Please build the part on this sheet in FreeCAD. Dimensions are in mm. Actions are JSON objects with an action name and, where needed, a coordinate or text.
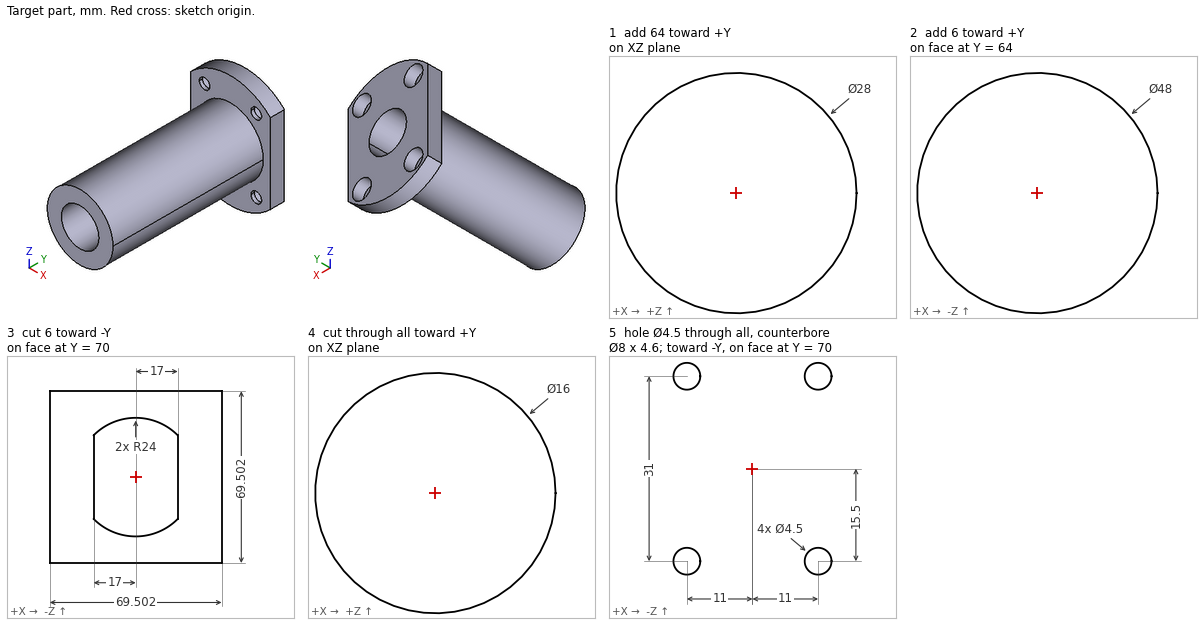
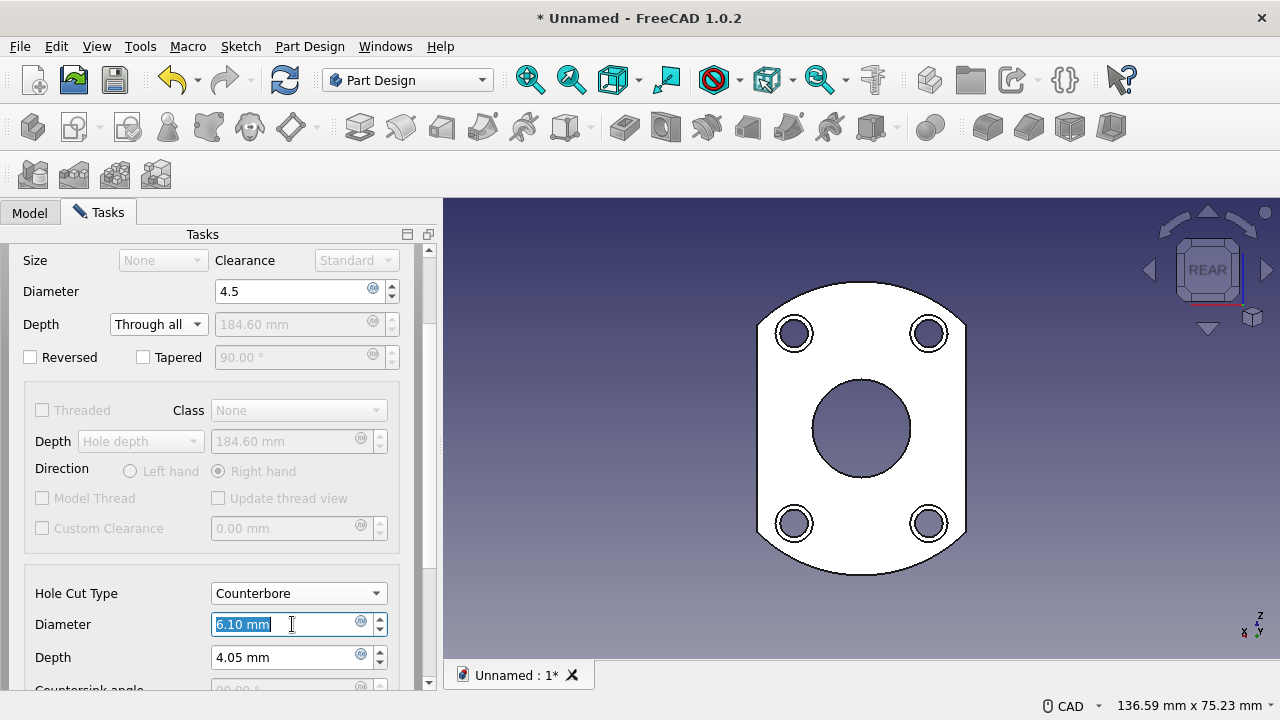
{"action": "type", "text": "8"}
{"action": "key", "text": "Tab"}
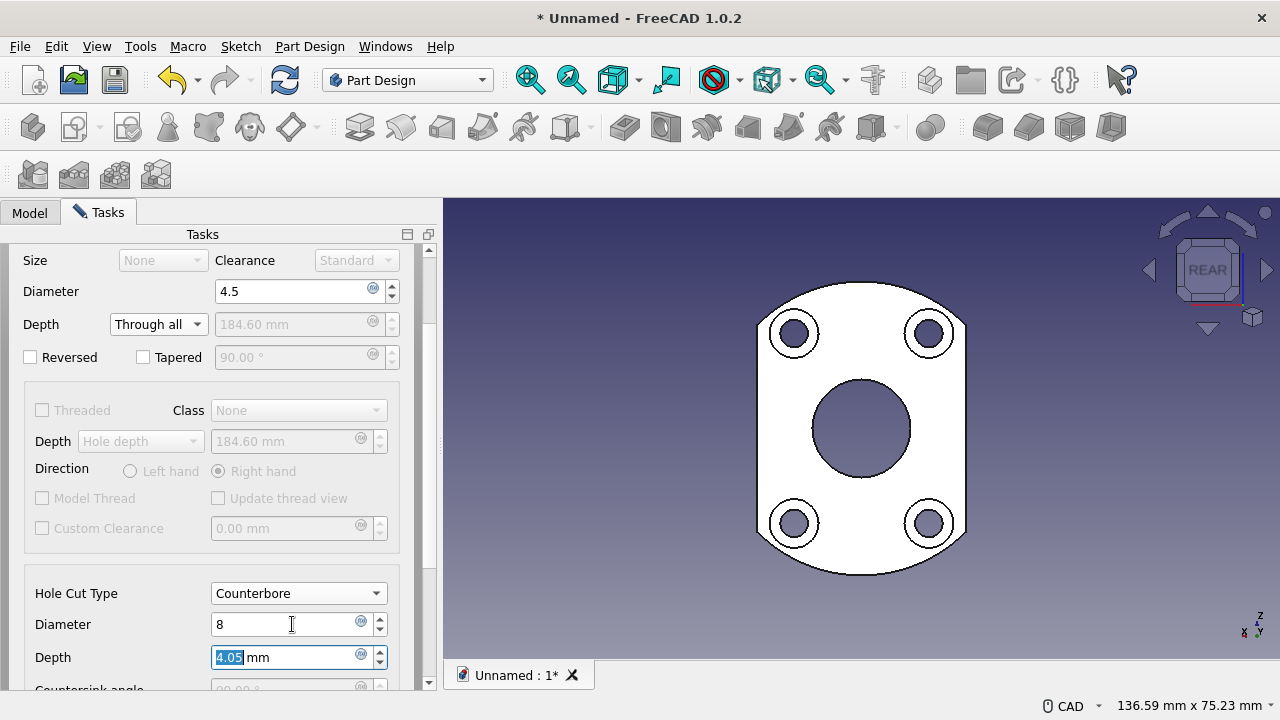
{"action": "type", "text": "4.6"}
{"action": "key", "text": "Tab"}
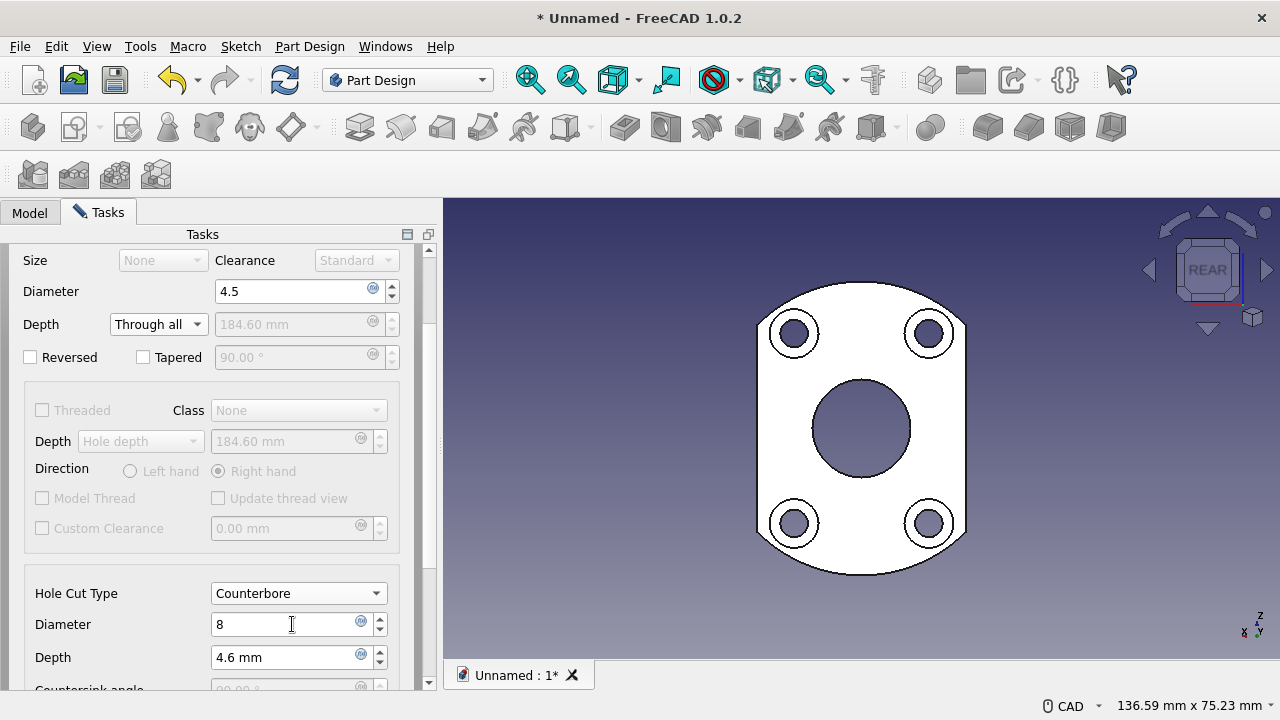
{"action": "scroll", "coordinate": [429, 467], "scroll_direction": "up", "scroll_amount": 3}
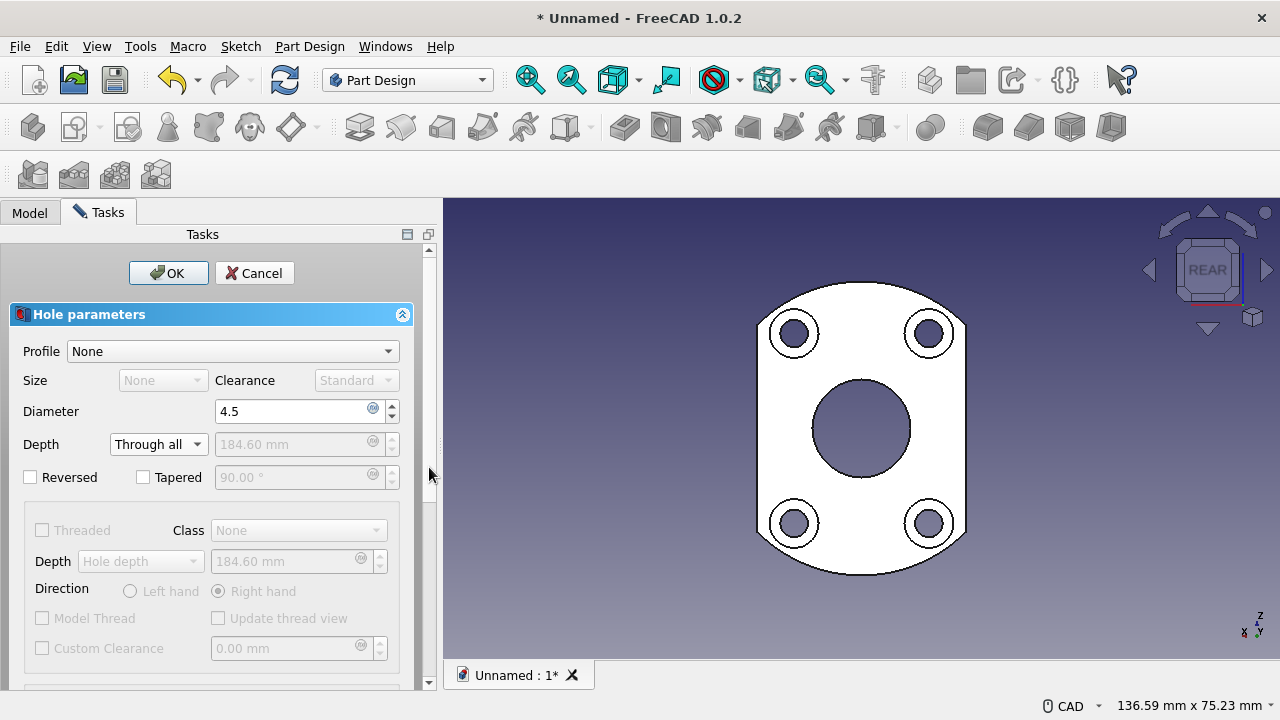
{"action": "left_click", "coordinate": [169, 273]}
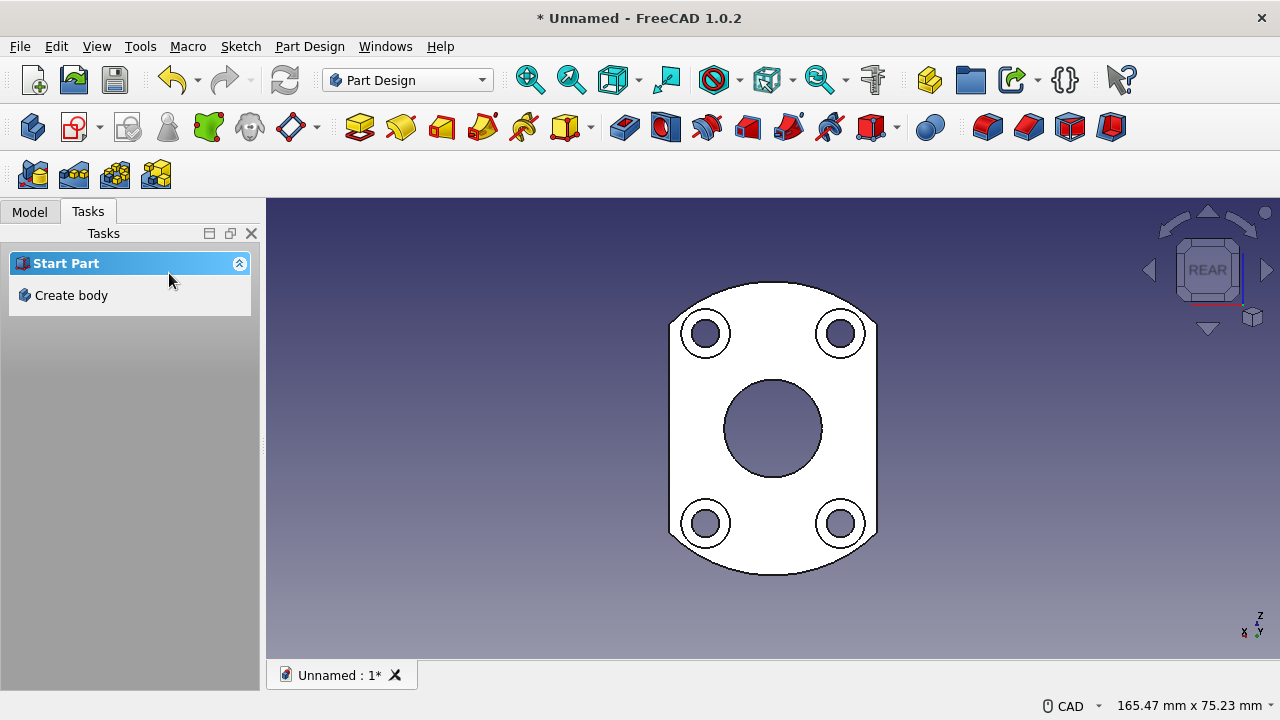
{"action": "key", "text": "0"}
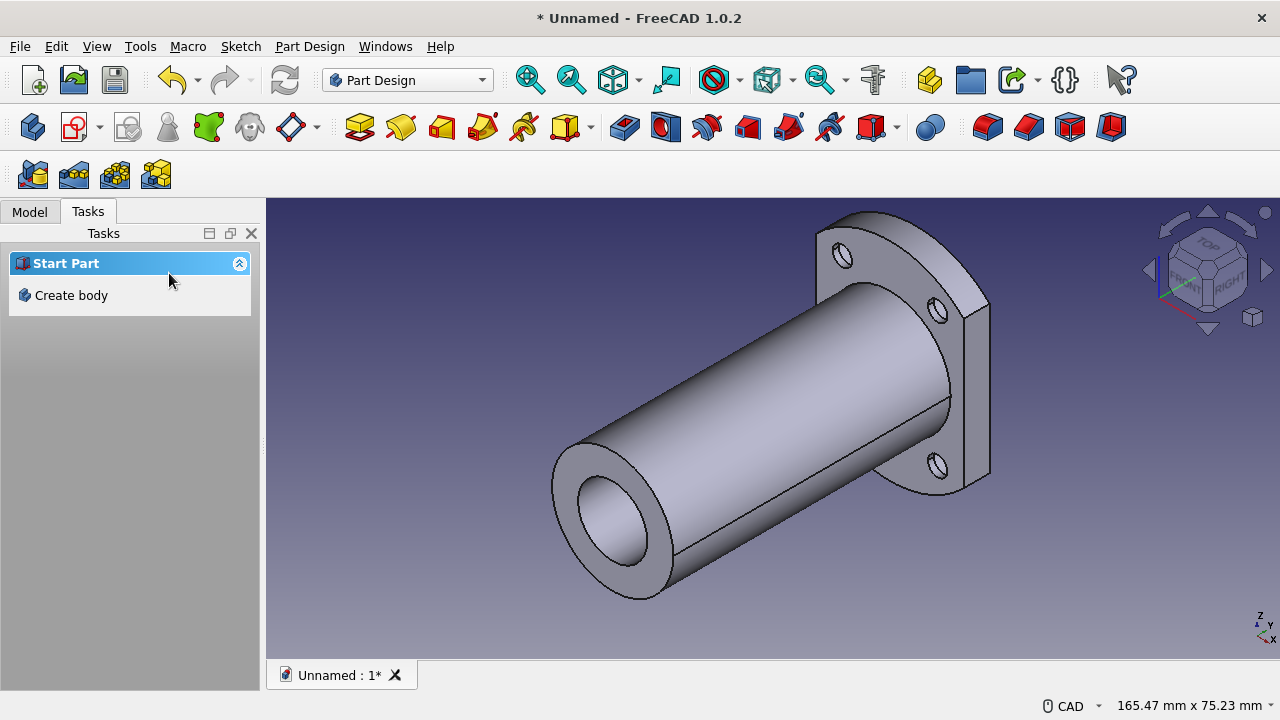
{"action": "left_click", "coordinate": [531, 80]}